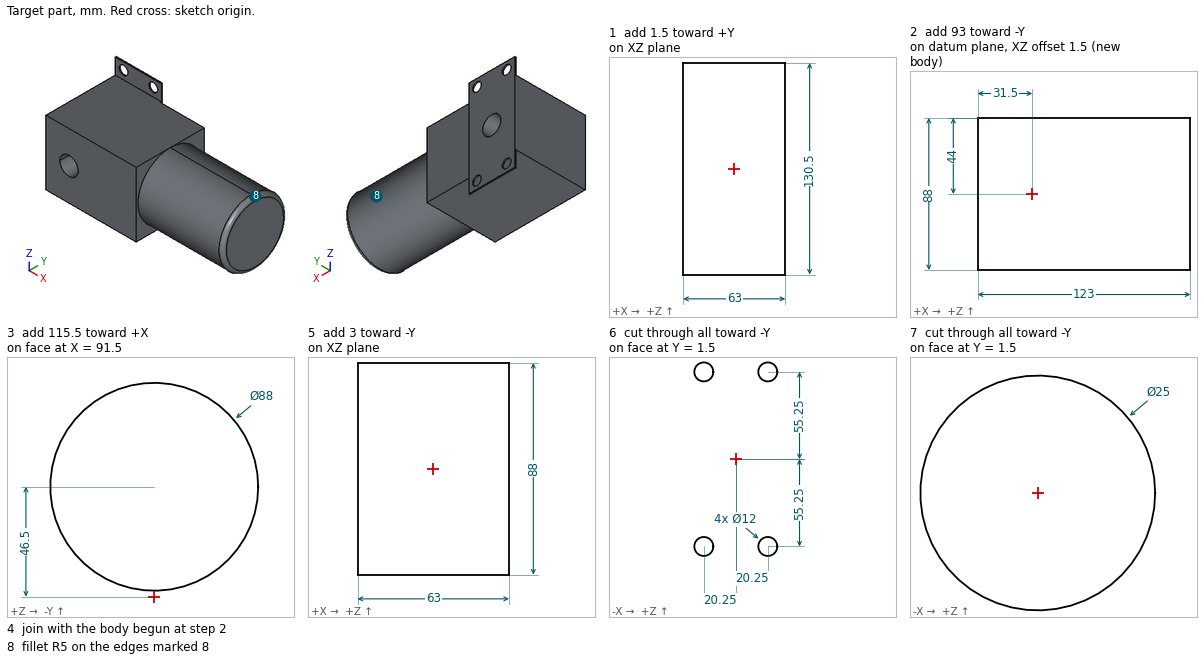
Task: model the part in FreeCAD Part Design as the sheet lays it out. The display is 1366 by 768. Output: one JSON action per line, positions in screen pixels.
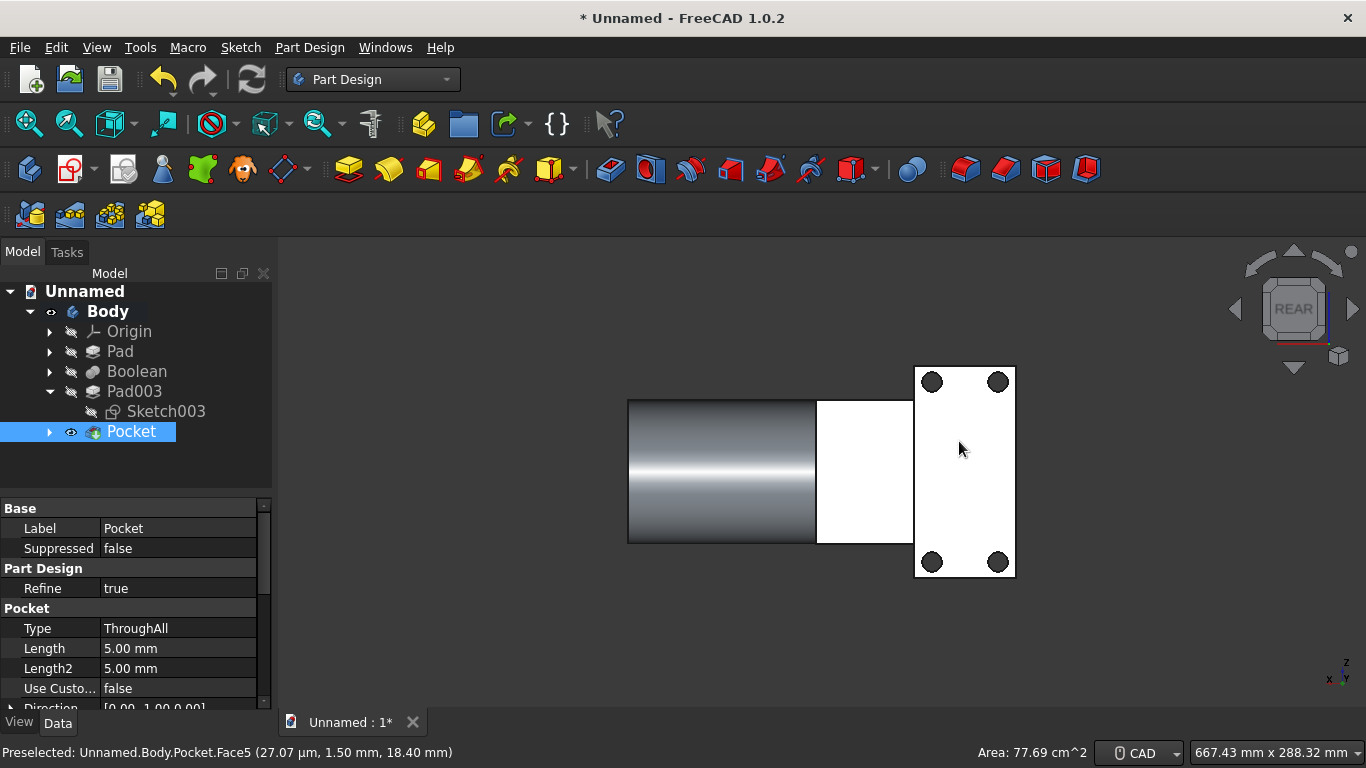
{"action": "left_click", "coordinate": [70, 170]}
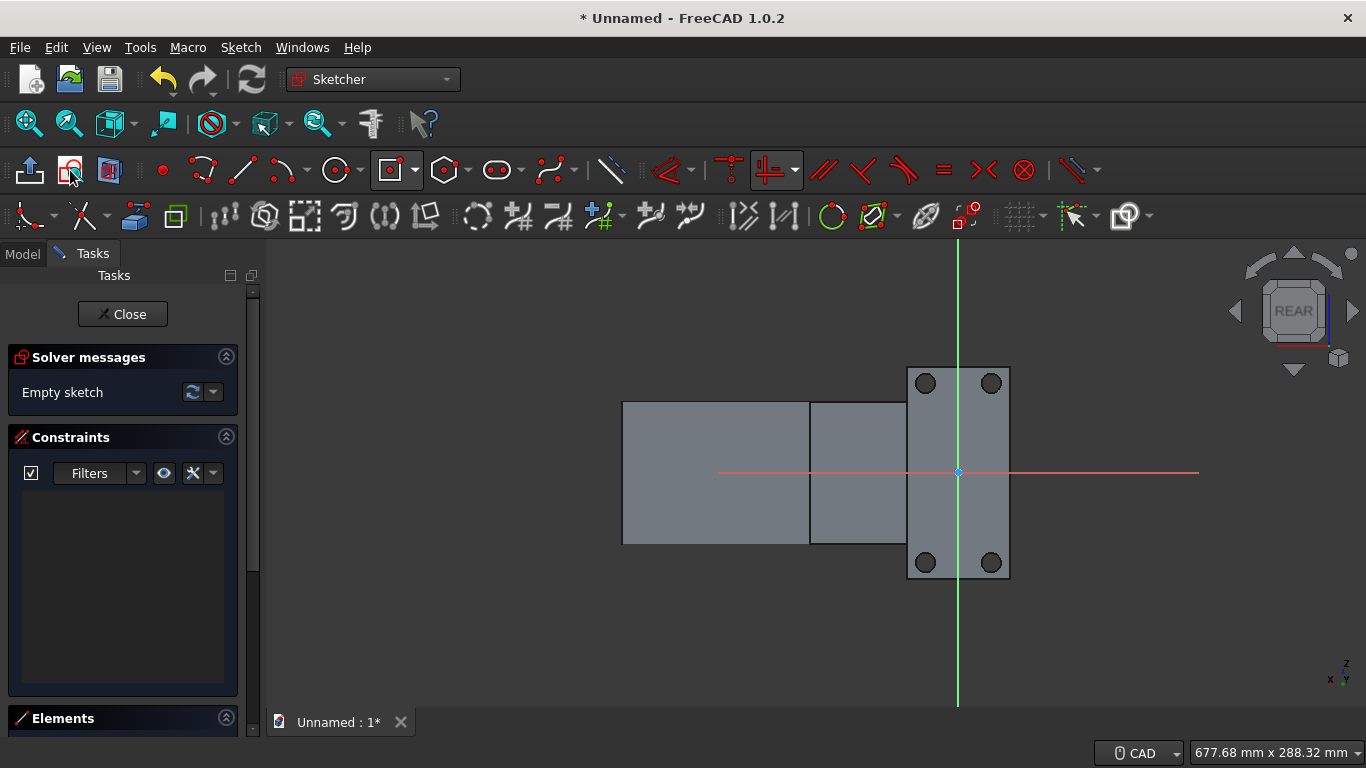
{"action": "scroll", "coordinate": [991, 473], "scroll_direction": "up", "scroll_amount": 10}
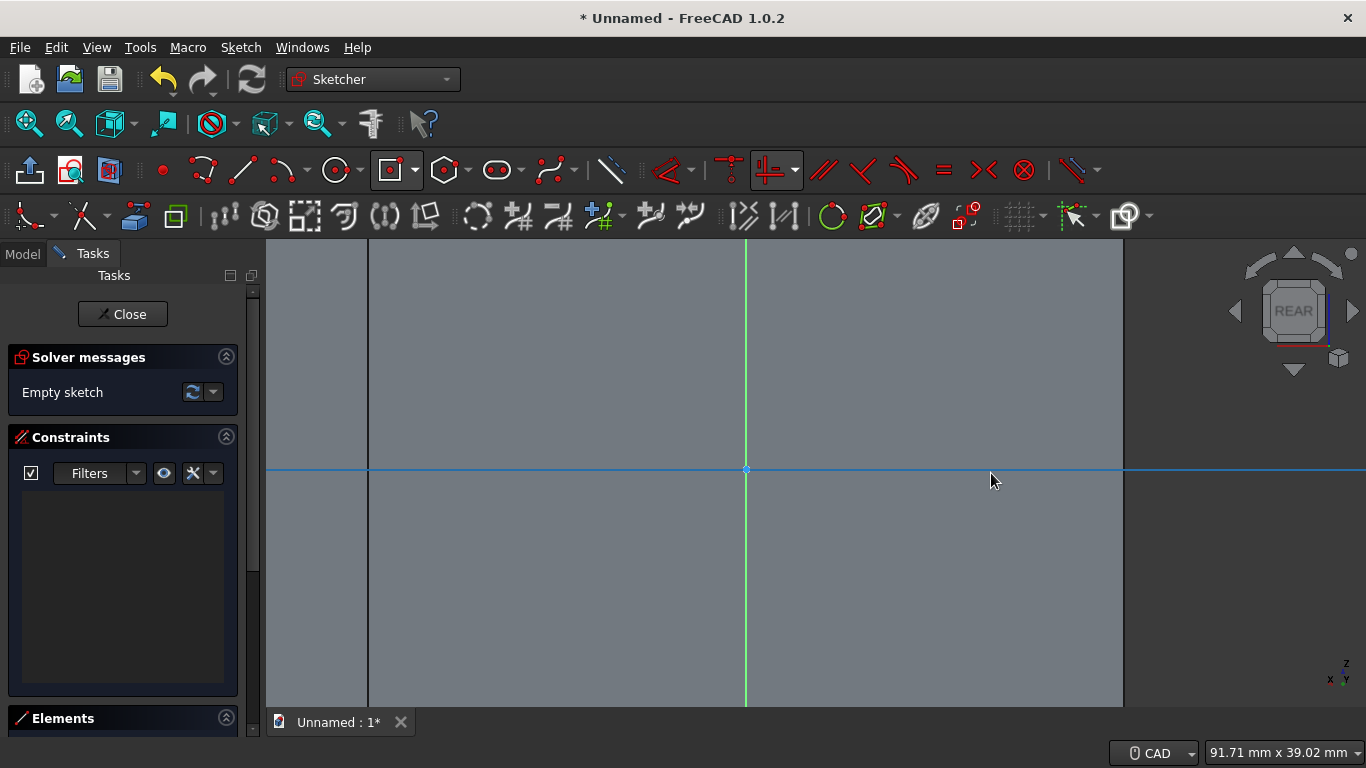
{"action": "left_click", "coordinate": [336, 170]}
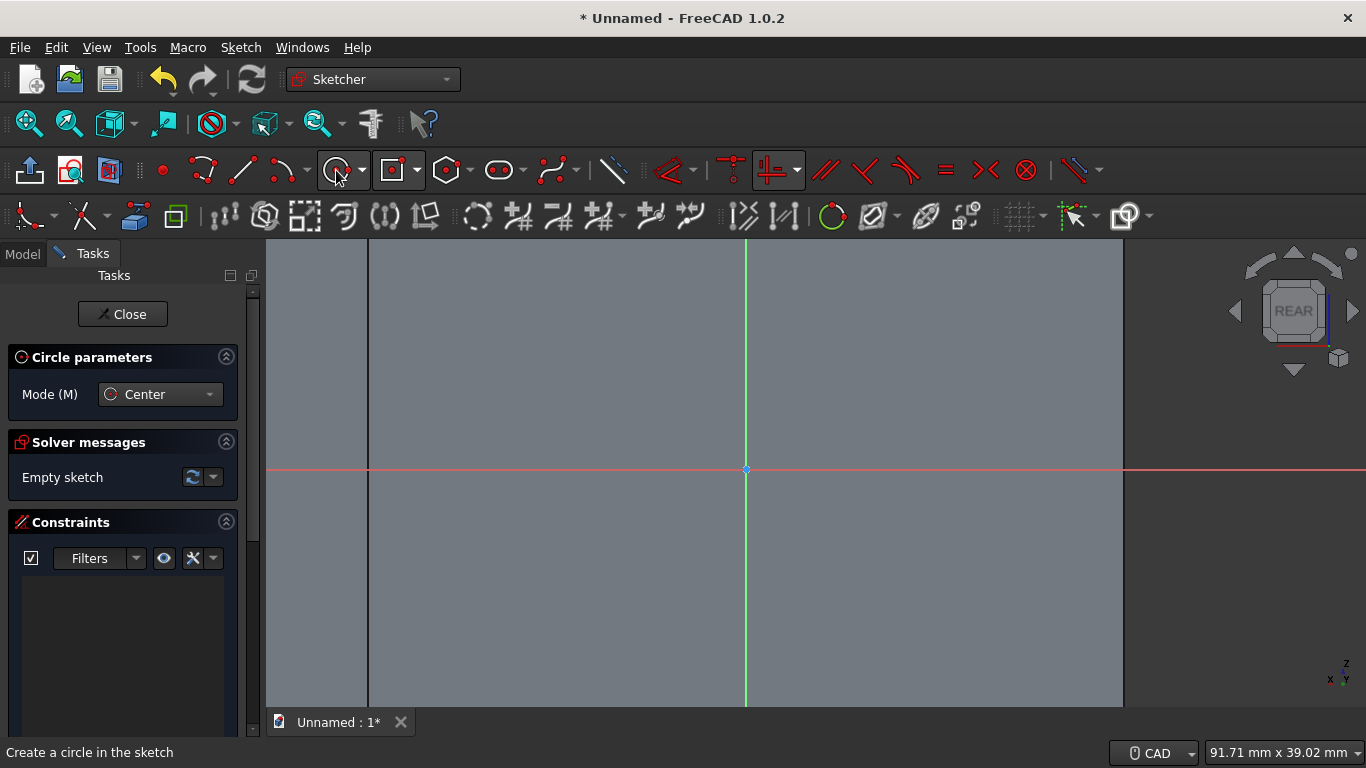
{"action": "left_click", "coordinate": [746, 470]}
{"action": "left_click", "coordinate": [852, 364]}
{"action": "key", "text": "Escape"}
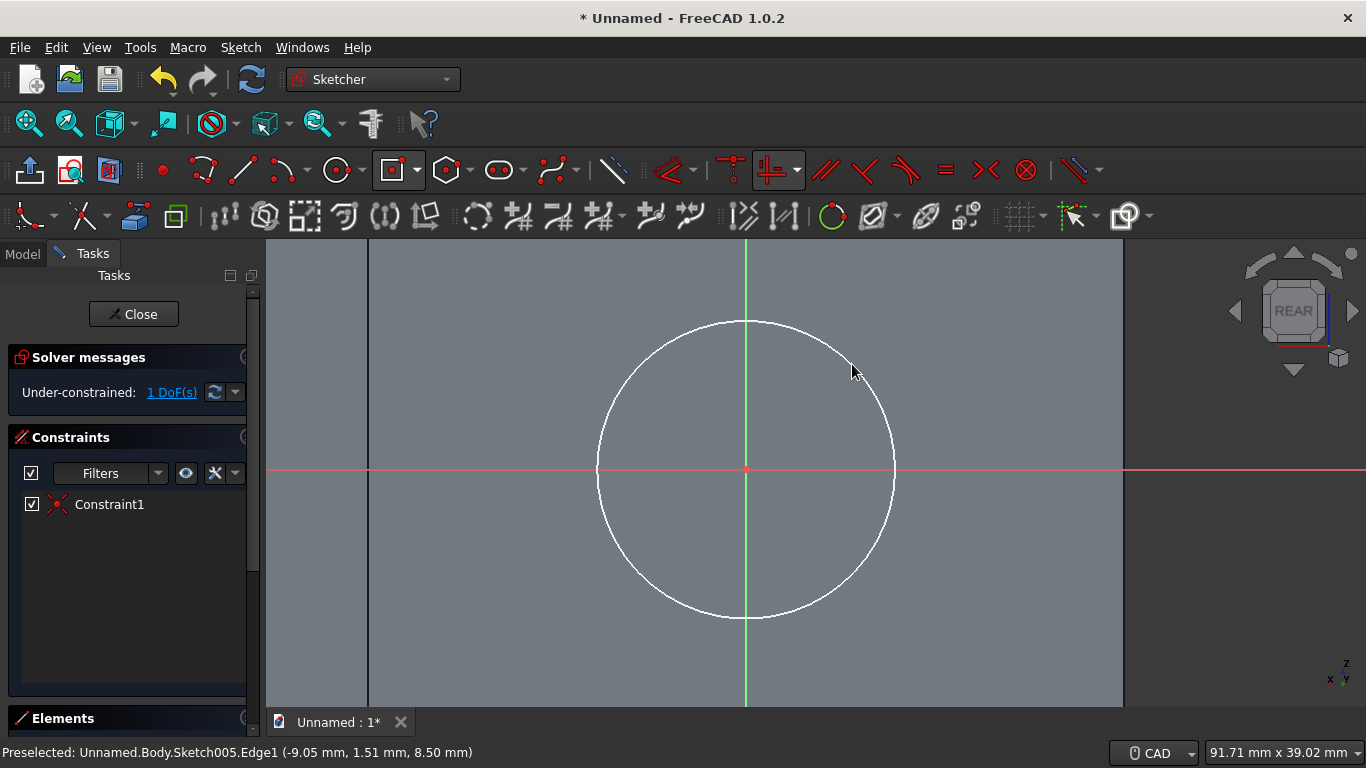
{"action": "left_click", "coordinate": [668, 170]}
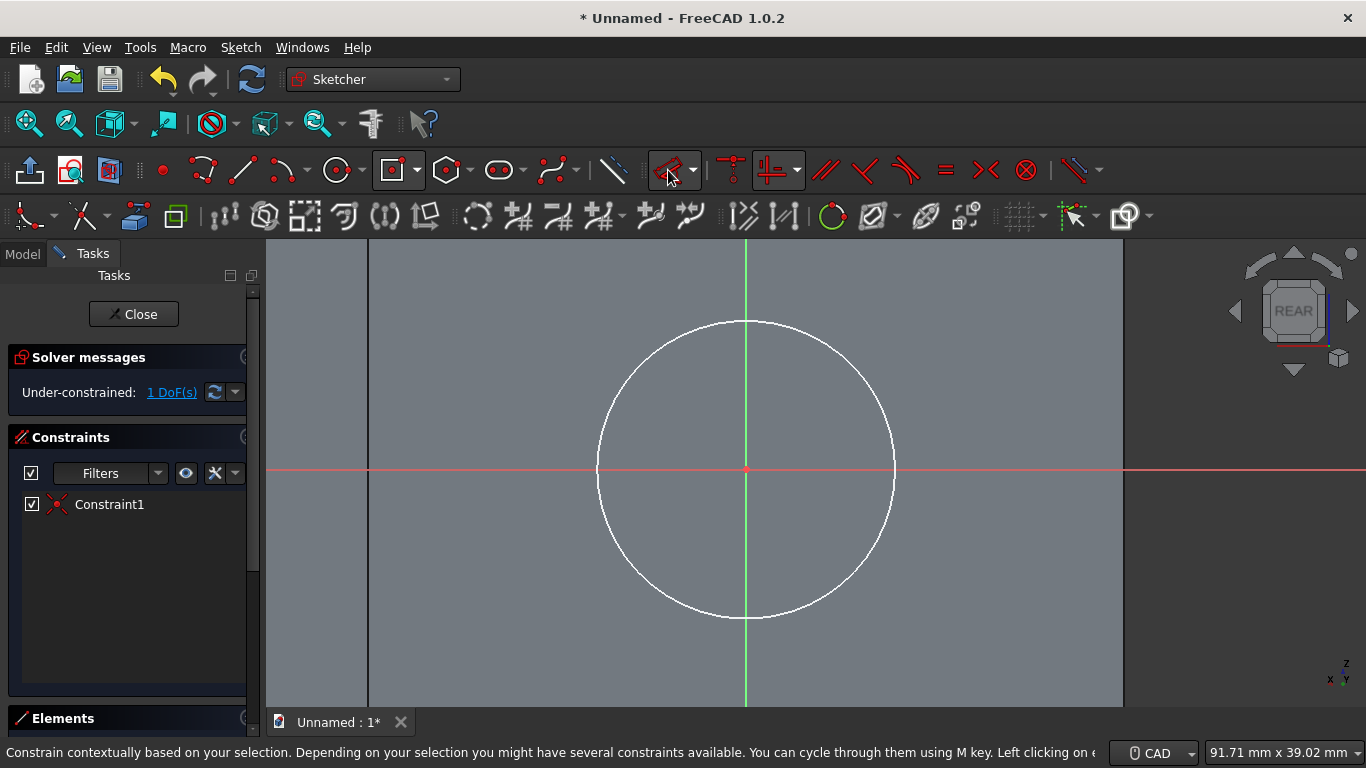
{"action": "left_click", "coordinate": [851, 364]}
{"action": "left_click", "coordinate": [874, 341]}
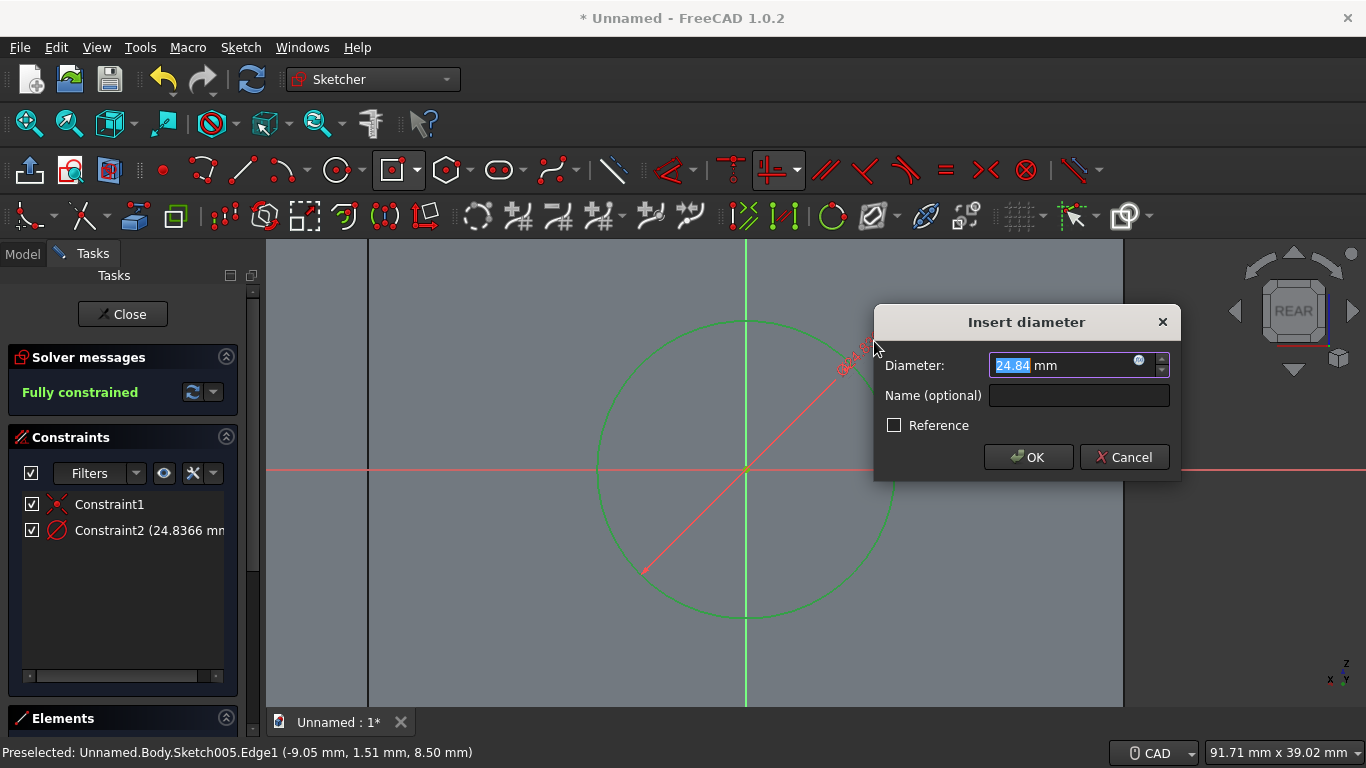
{"action": "type", "text": "25"}
{"action": "key", "text": "Return"}
{"action": "key", "text": "Escape"}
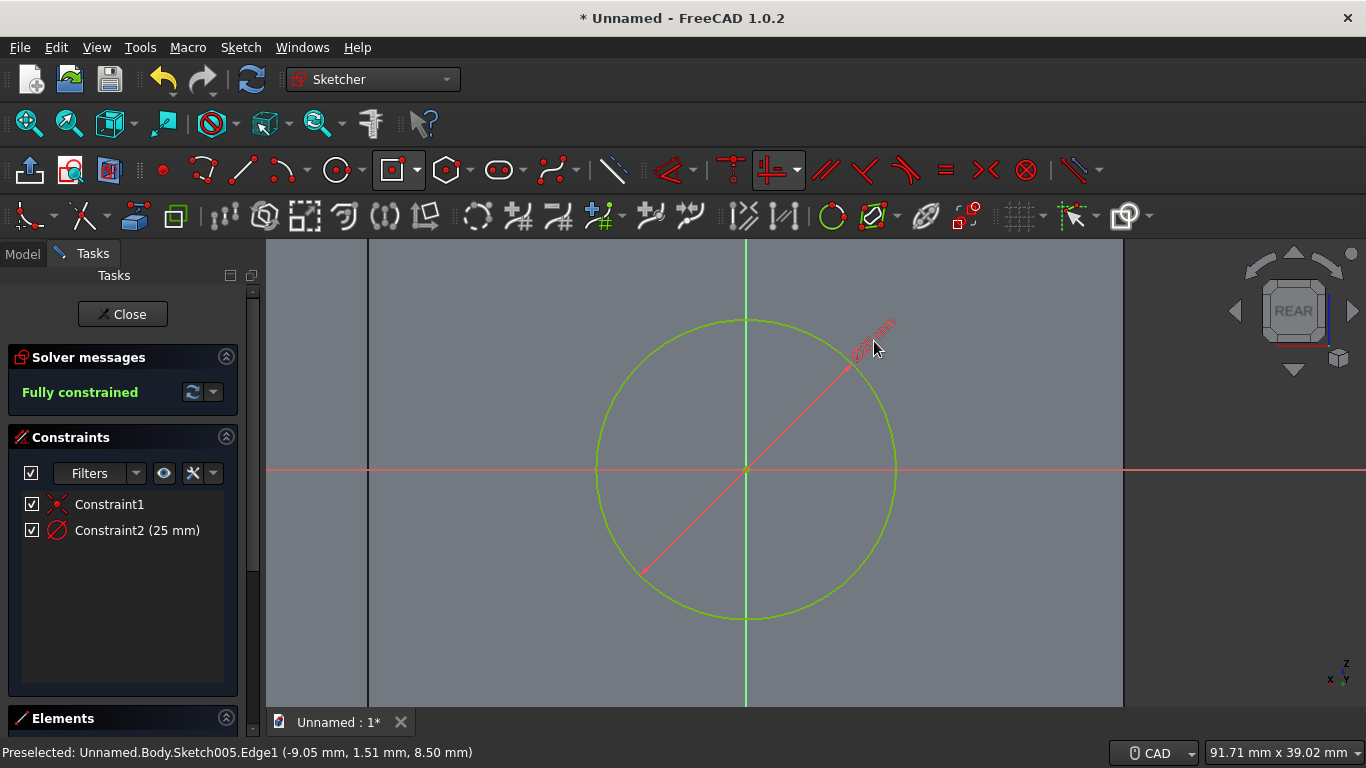
{"action": "left_click", "coordinate": [123, 314]}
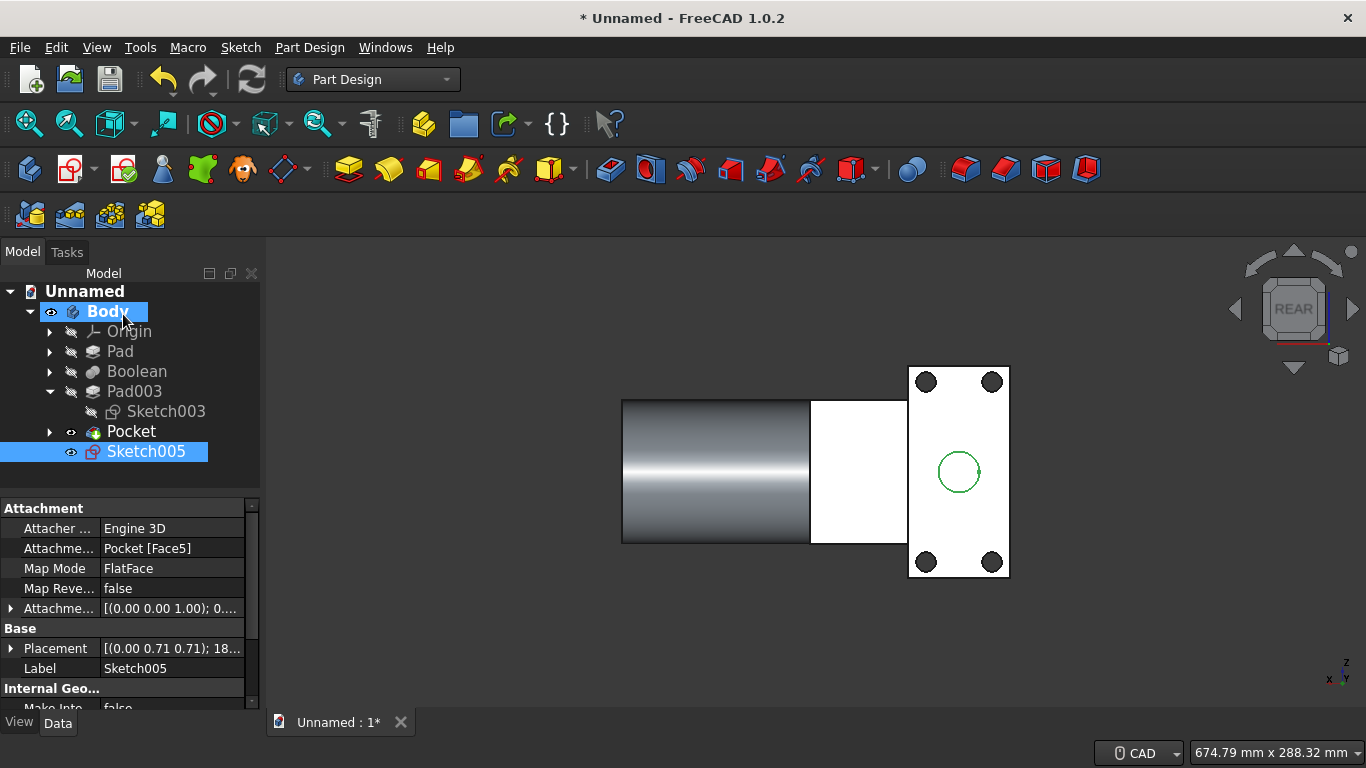
{"action": "left_click", "coordinate": [612, 170]}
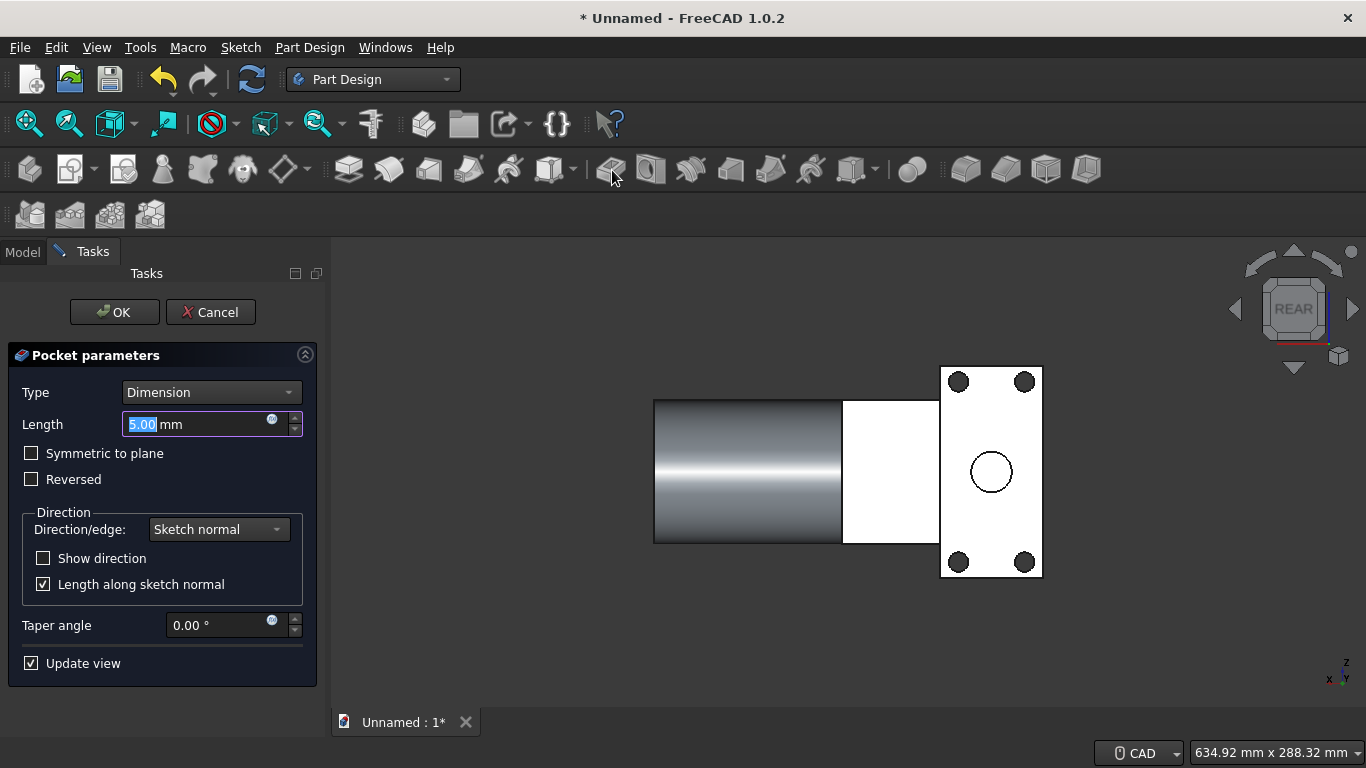
{"action": "left_click", "coordinate": [212, 392]}